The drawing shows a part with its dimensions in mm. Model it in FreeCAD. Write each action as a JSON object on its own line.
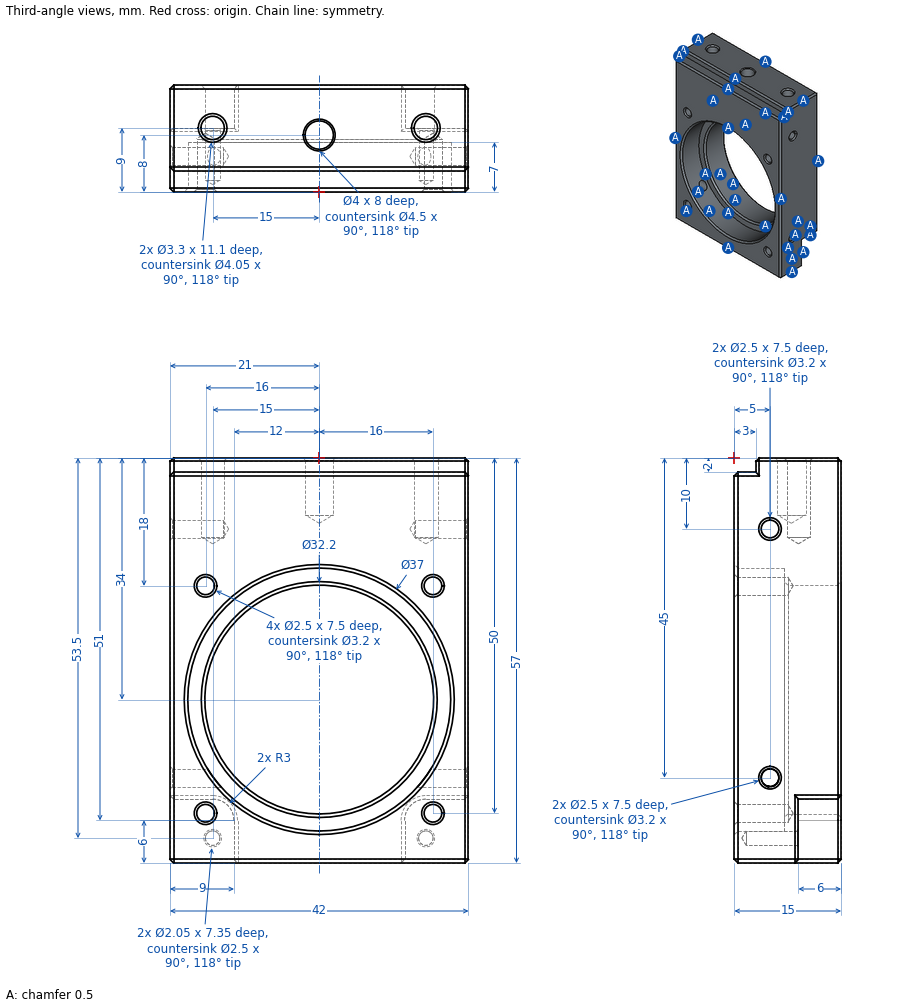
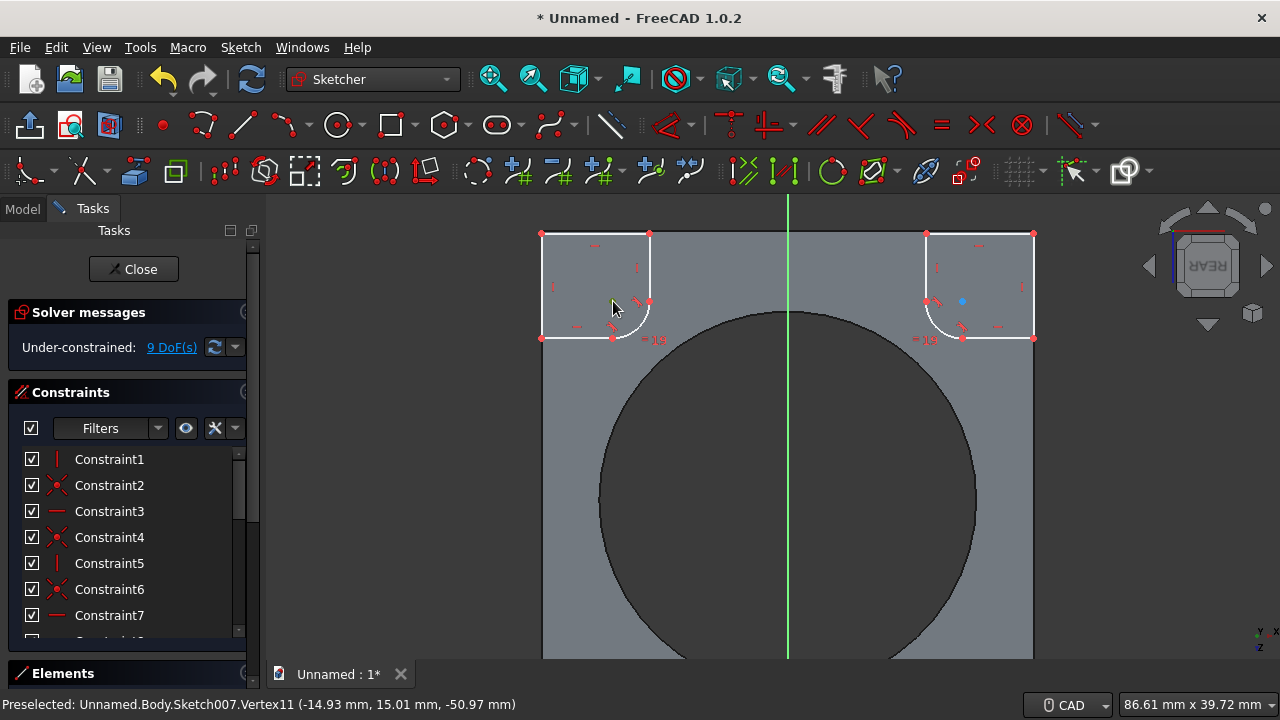
{"action": "left_click", "coordinate": [963, 302]}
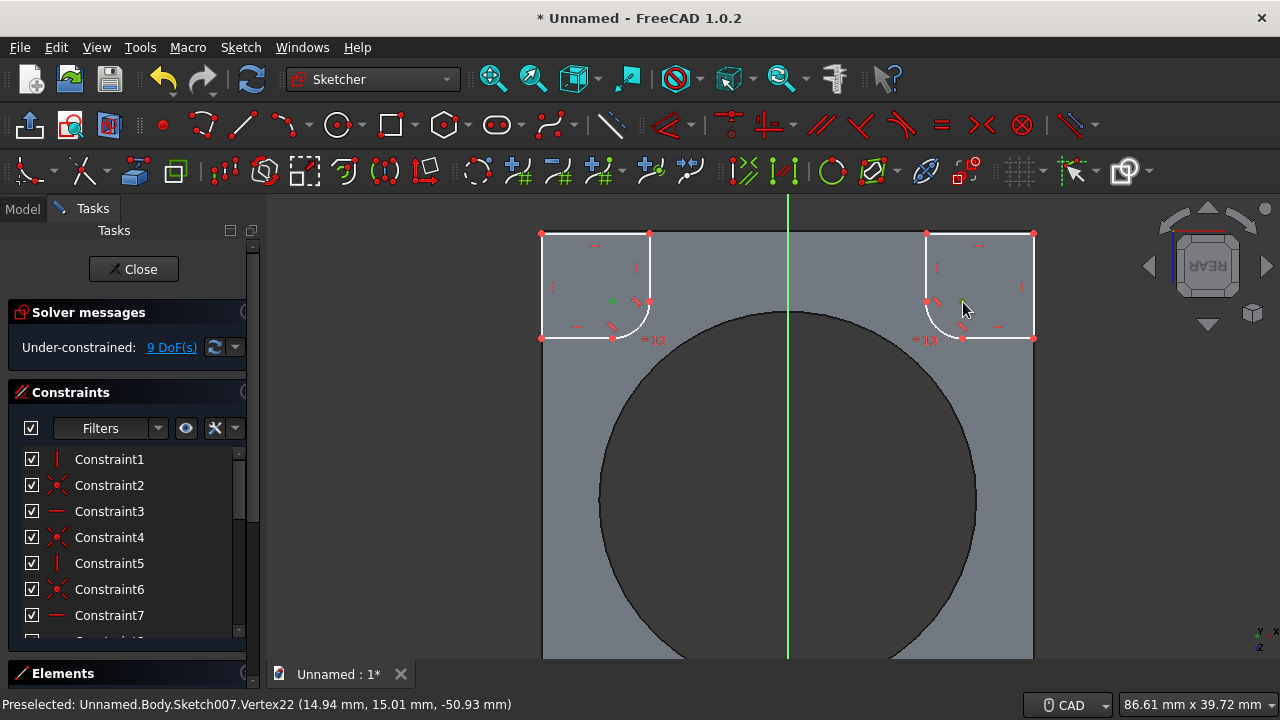
{"action": "left_click", "coordinate": [788, 602]}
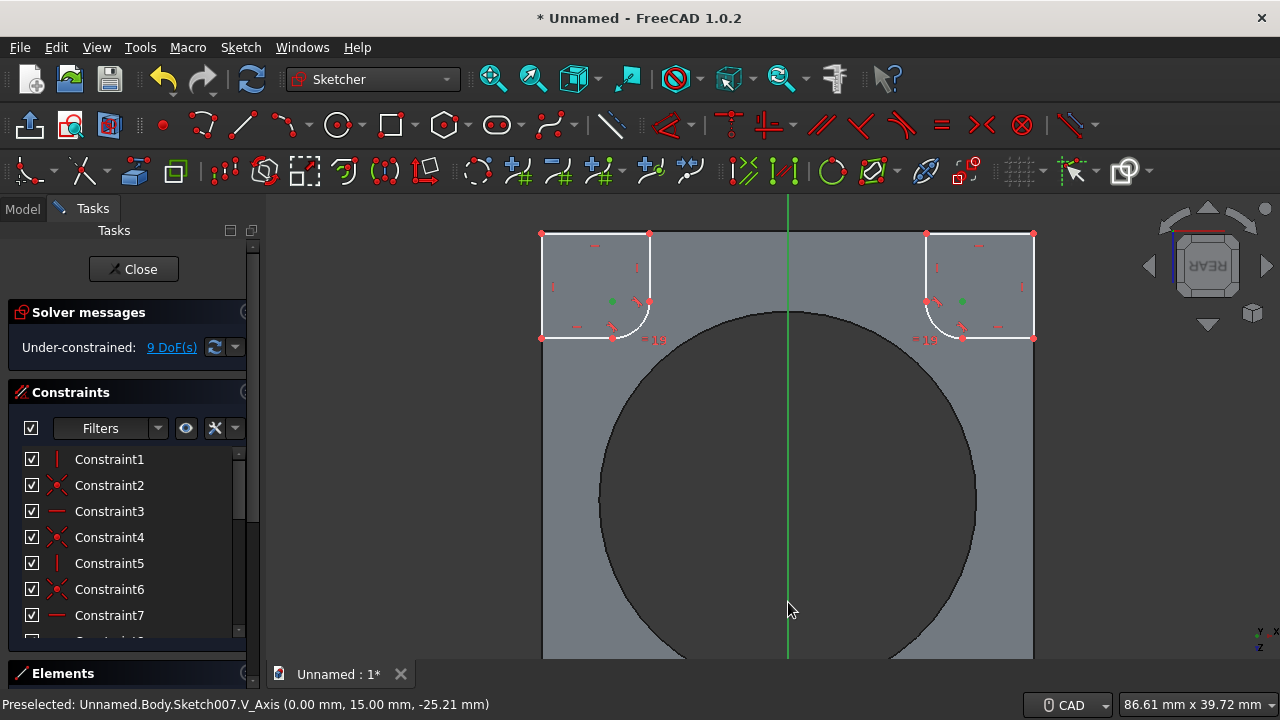
{"action": "left_click", "coordinate": [982, 126]}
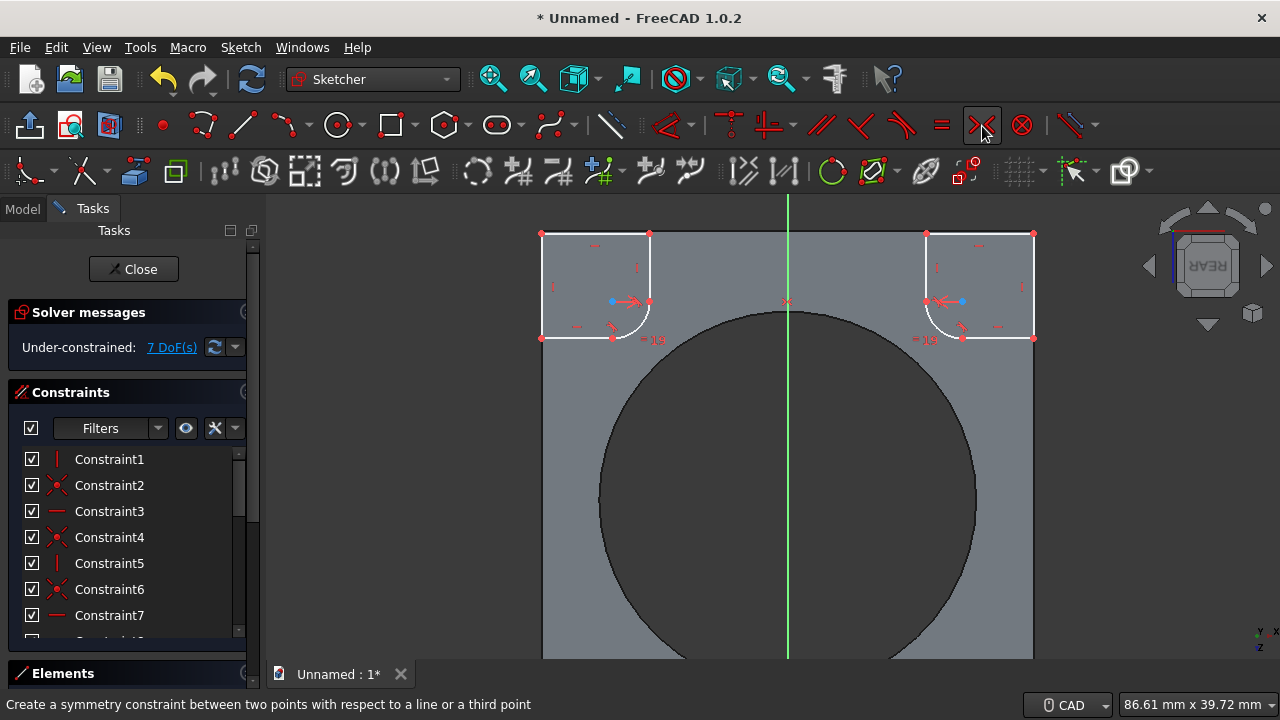
{"action": "left_click", "coordinate": [542, 234]}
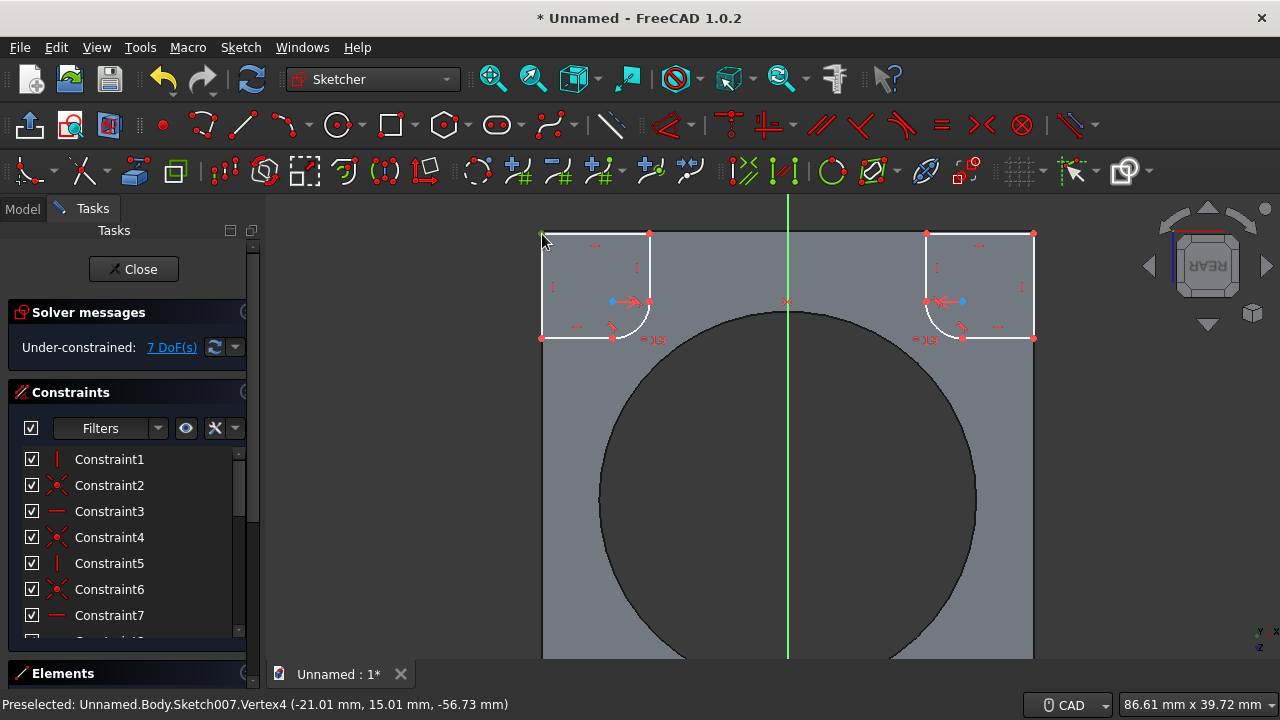
{"action": "left_click", "coordinate": [1034, 234]}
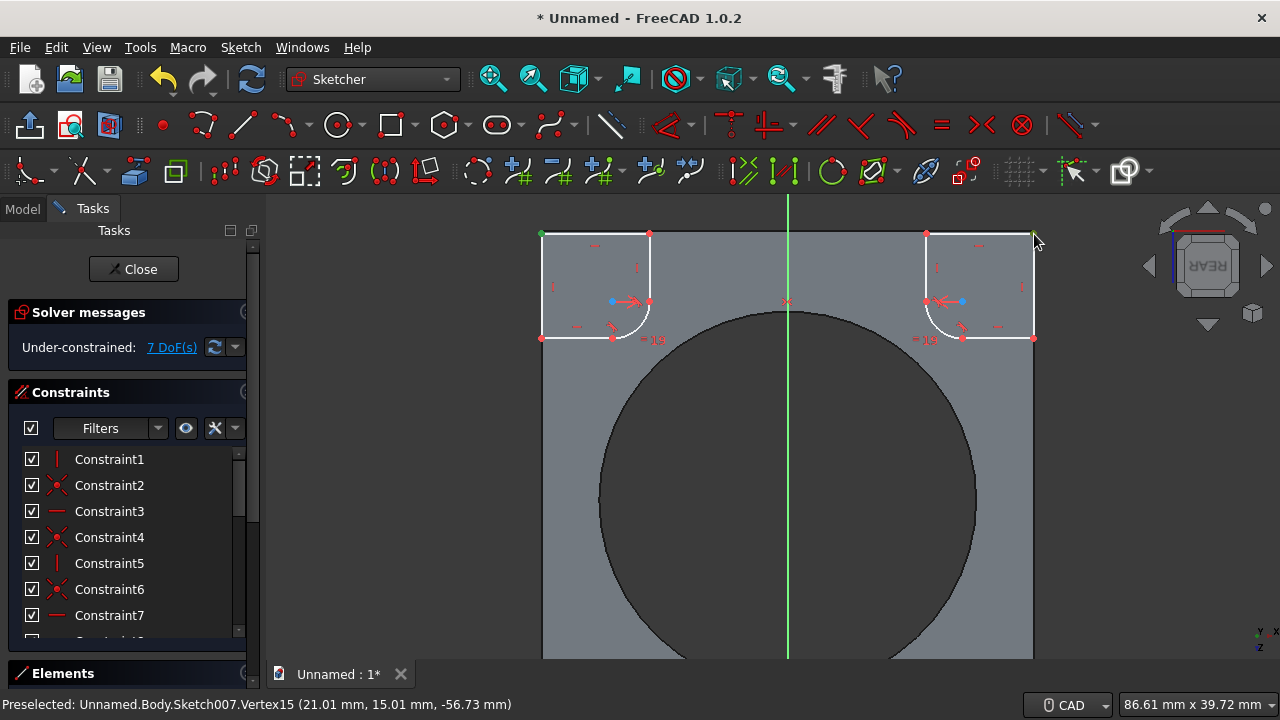
{"action": "left_click", "coordinate": [788, 602]}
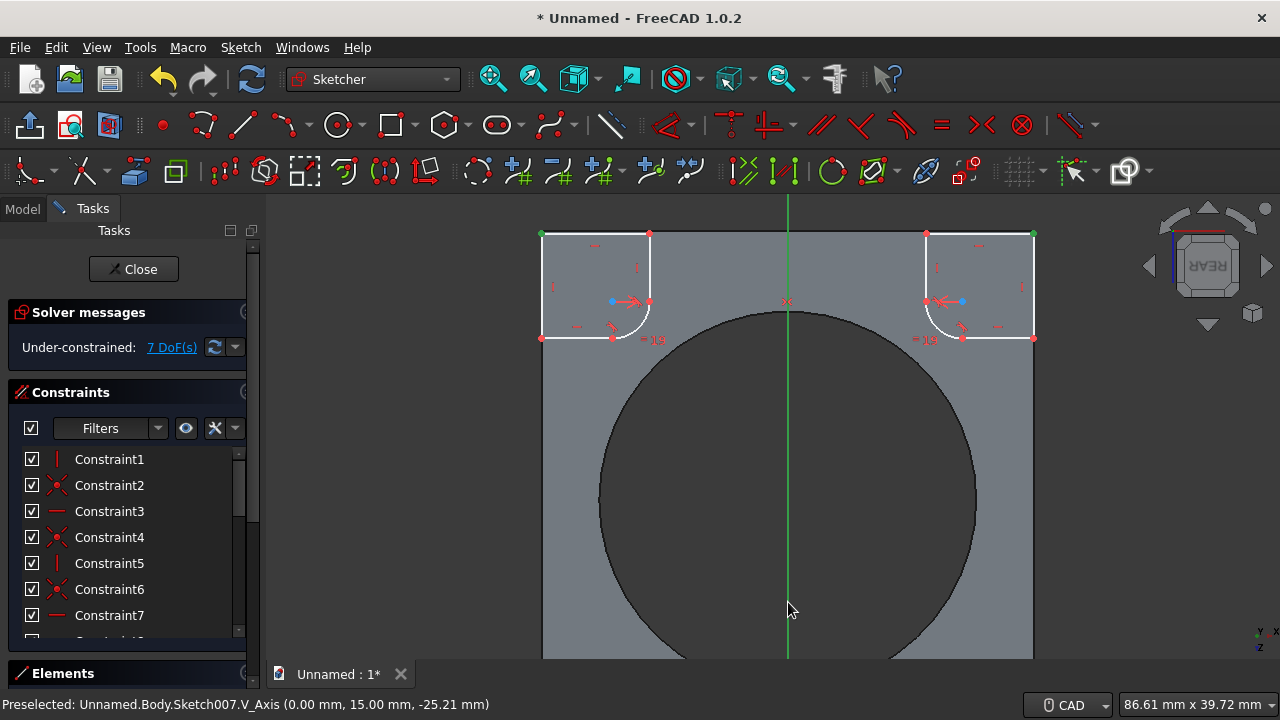
{"action": "left_click", "coordinate": [982, 126]}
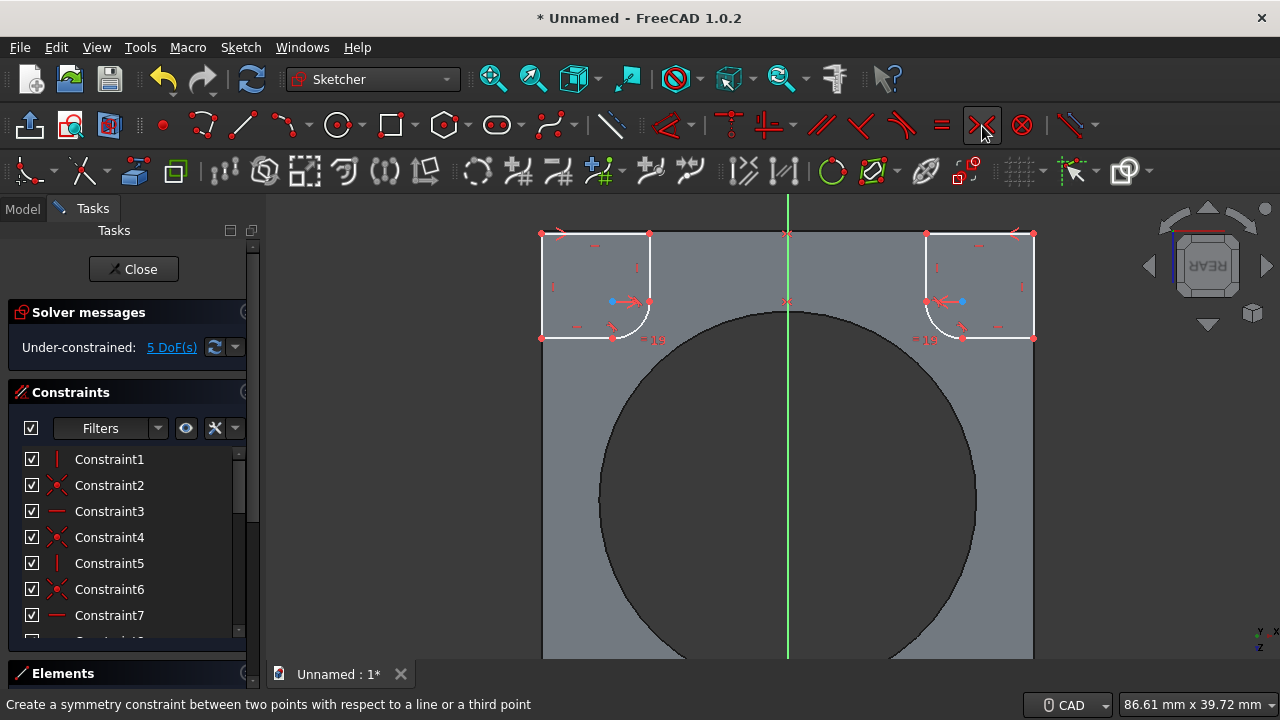
{"action": "key", "text": "d"}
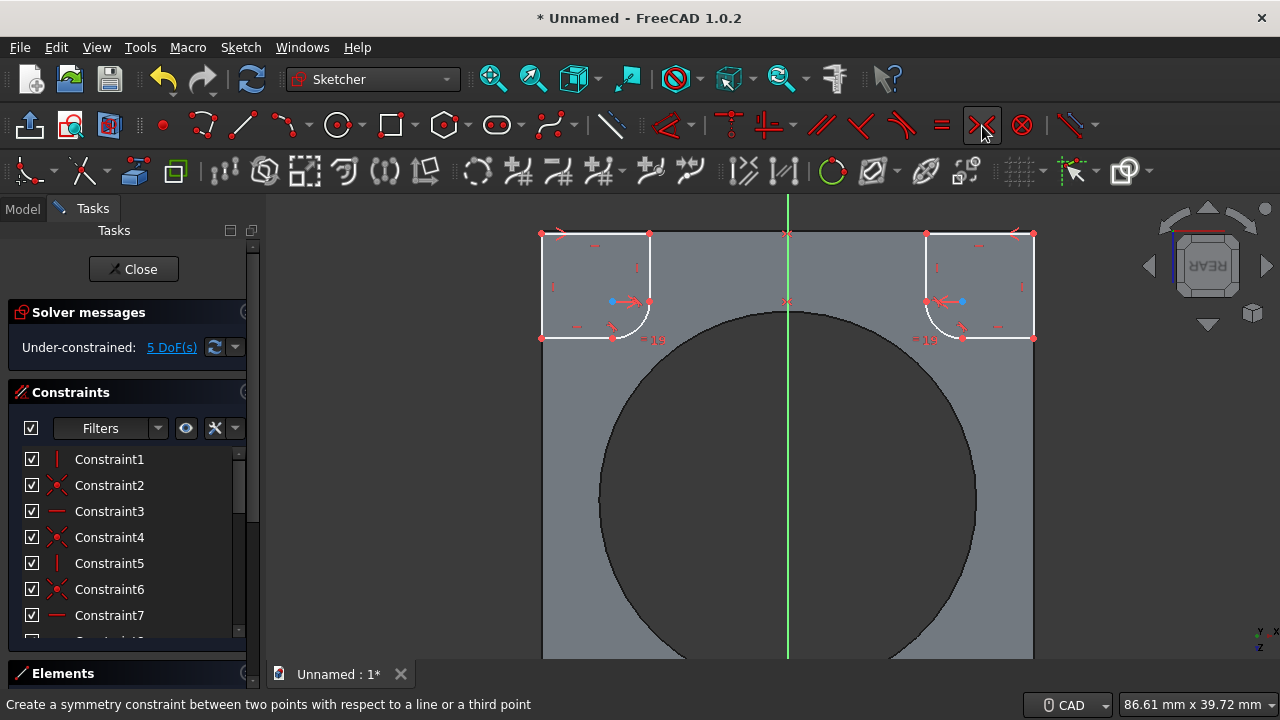
{"action": "left_click", "coordinate": [630, 334]}
{"action": "left_click", "coordinate": [645, 362]}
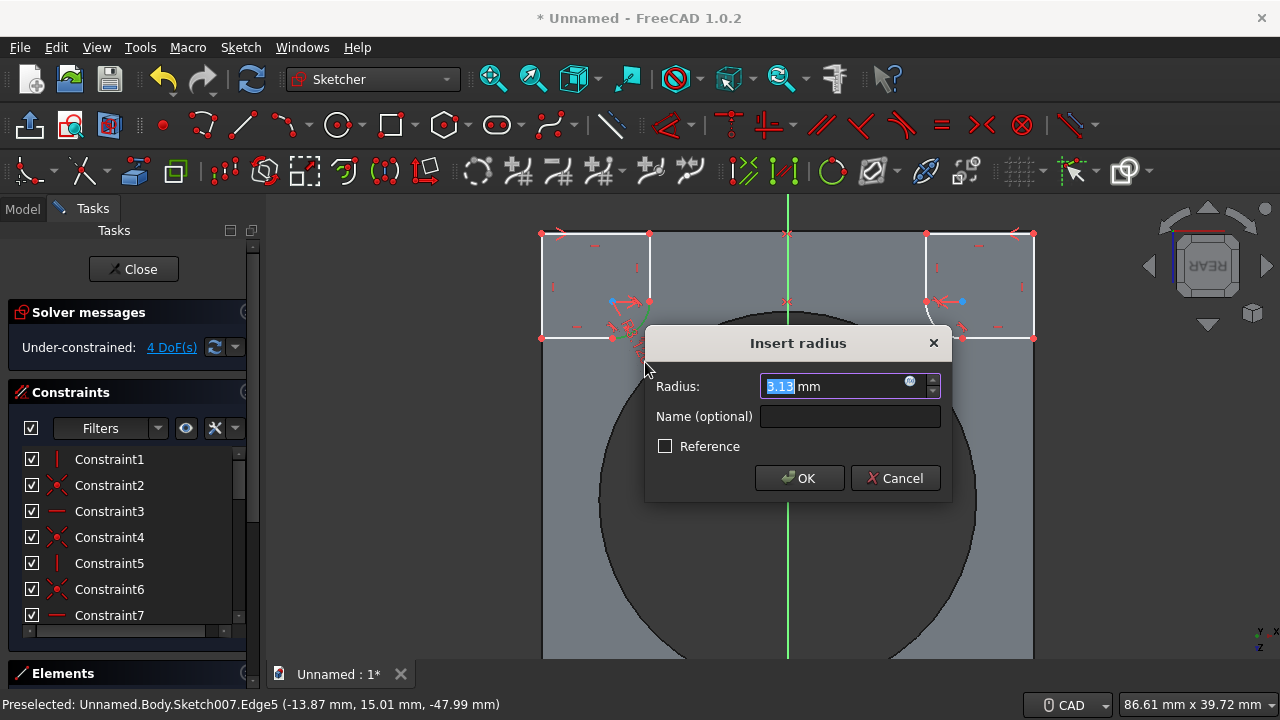
{"action": "type", "text": "3"}
{"action": "key", "text": "Return"}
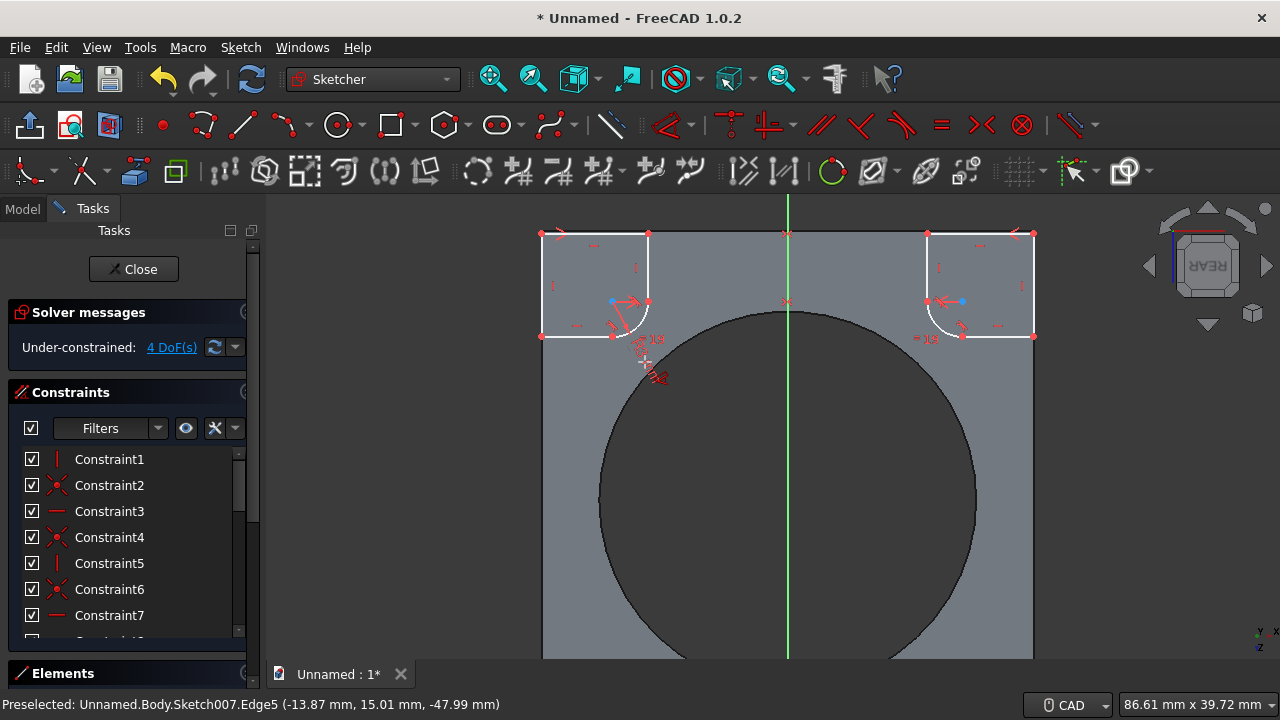
{"action": "left_click", "coordinate": [648, 281]}
{"action": "left_click", "coordinate": [614, 268]}